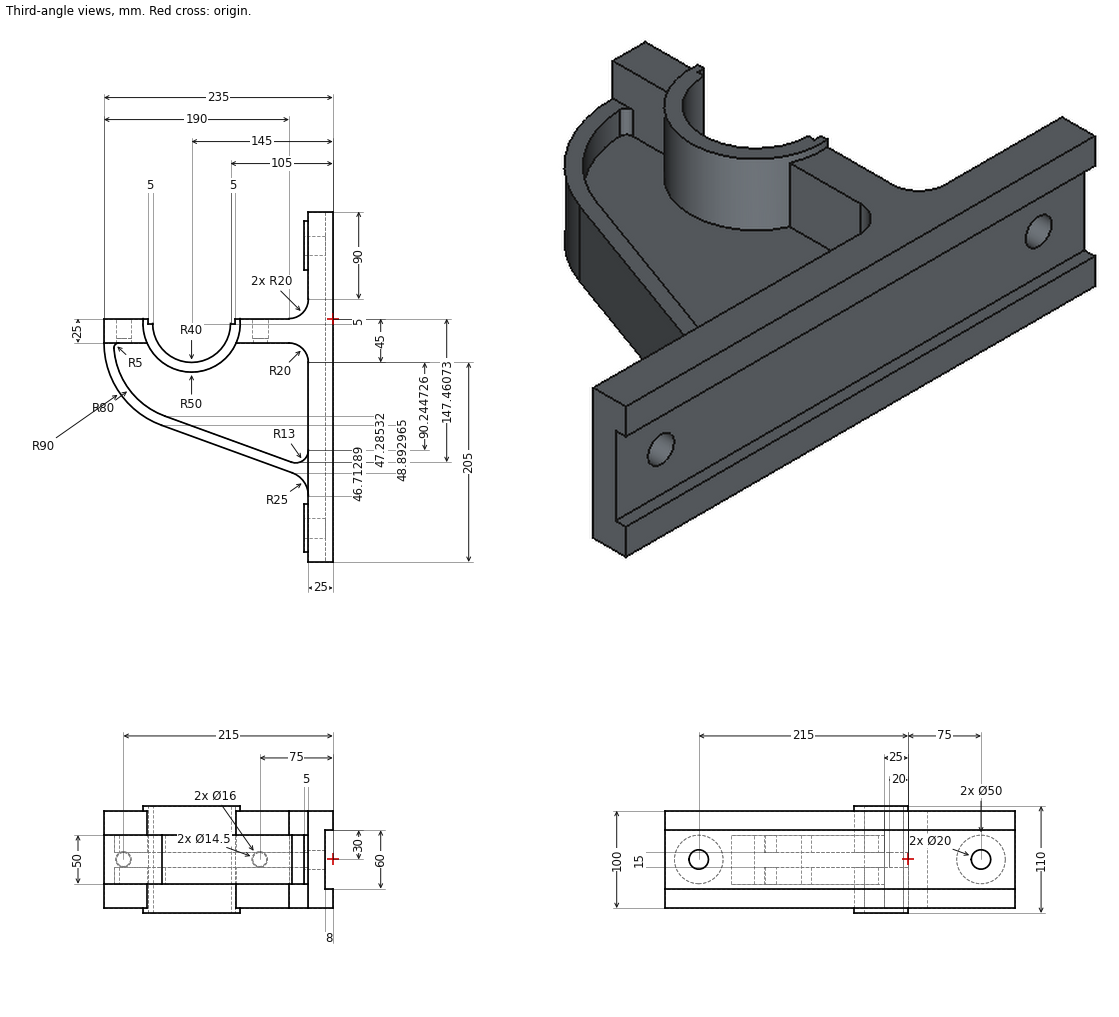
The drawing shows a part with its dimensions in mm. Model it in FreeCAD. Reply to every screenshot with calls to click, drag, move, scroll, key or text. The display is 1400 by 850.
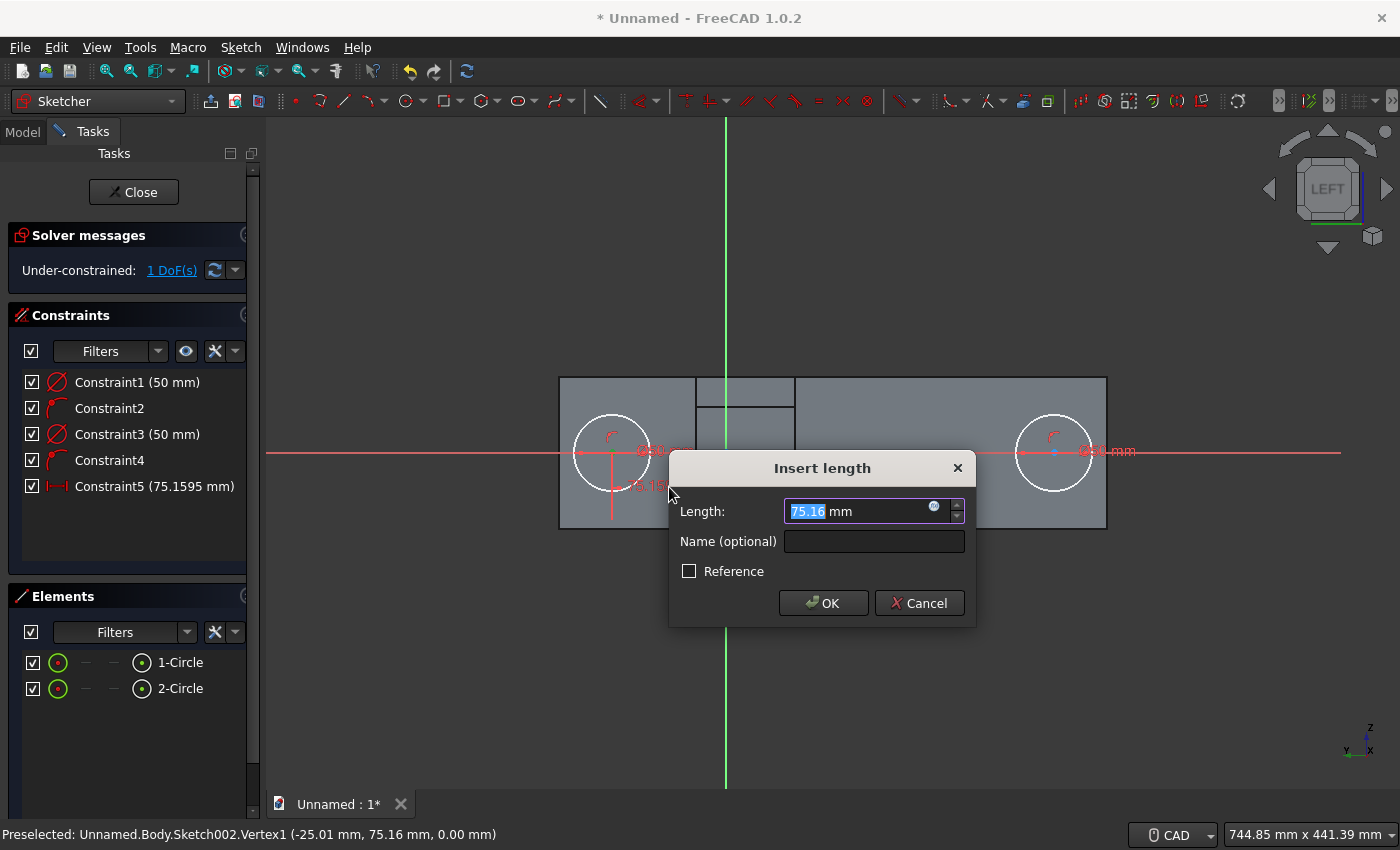
text(75)
key(Return)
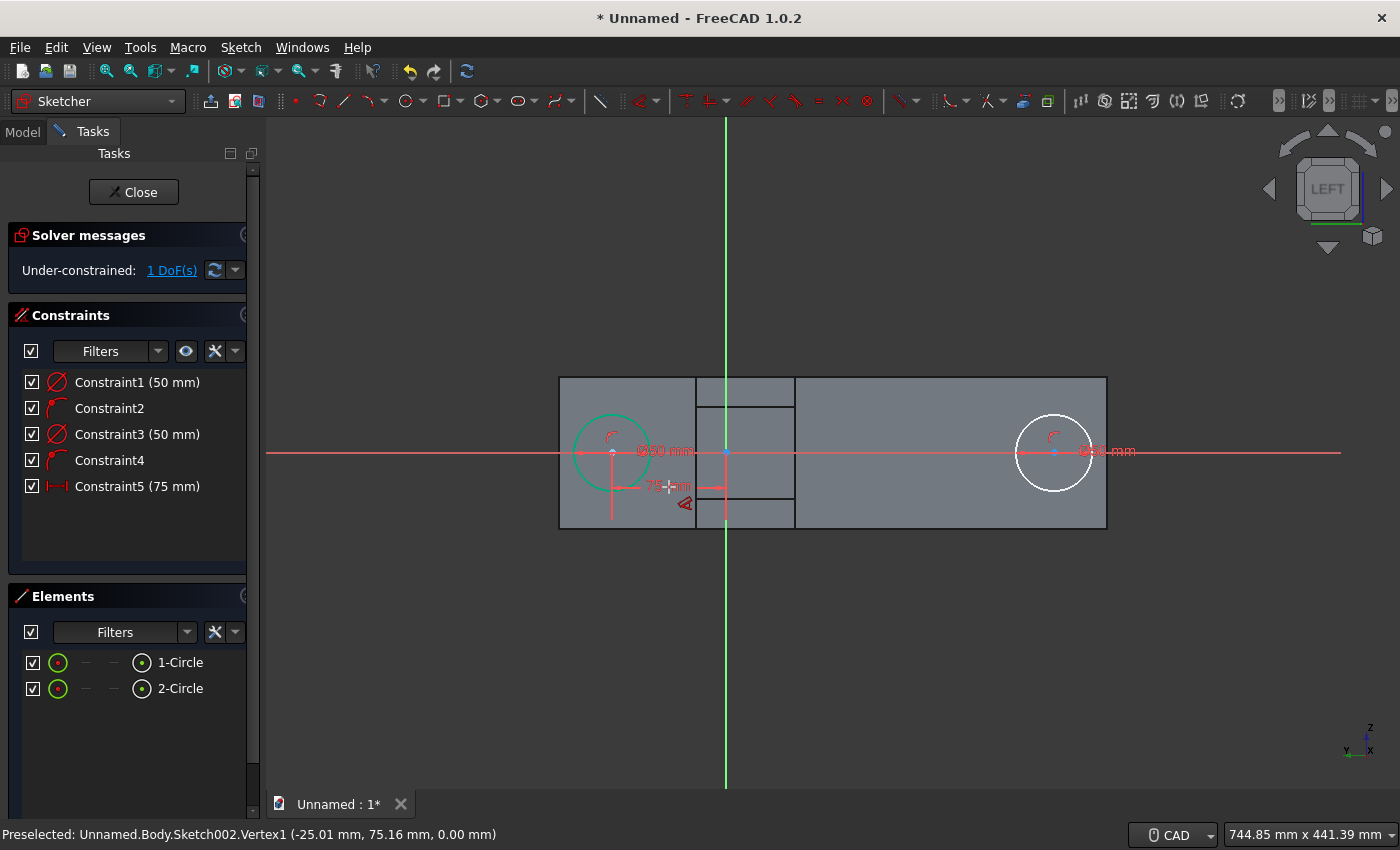
click(1054, 453)
click(890, 487)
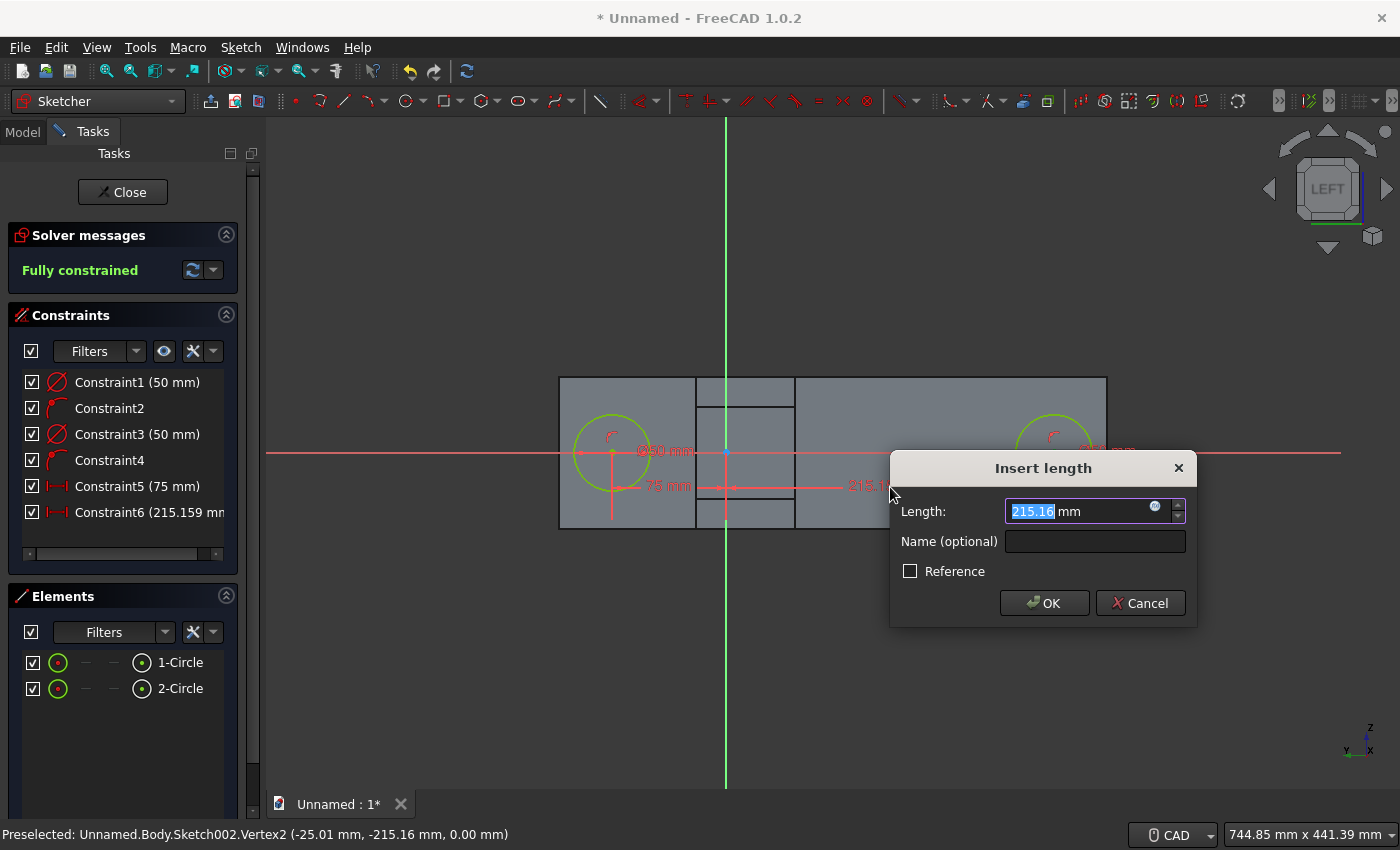
text(215)
key(Return)
key(Escape)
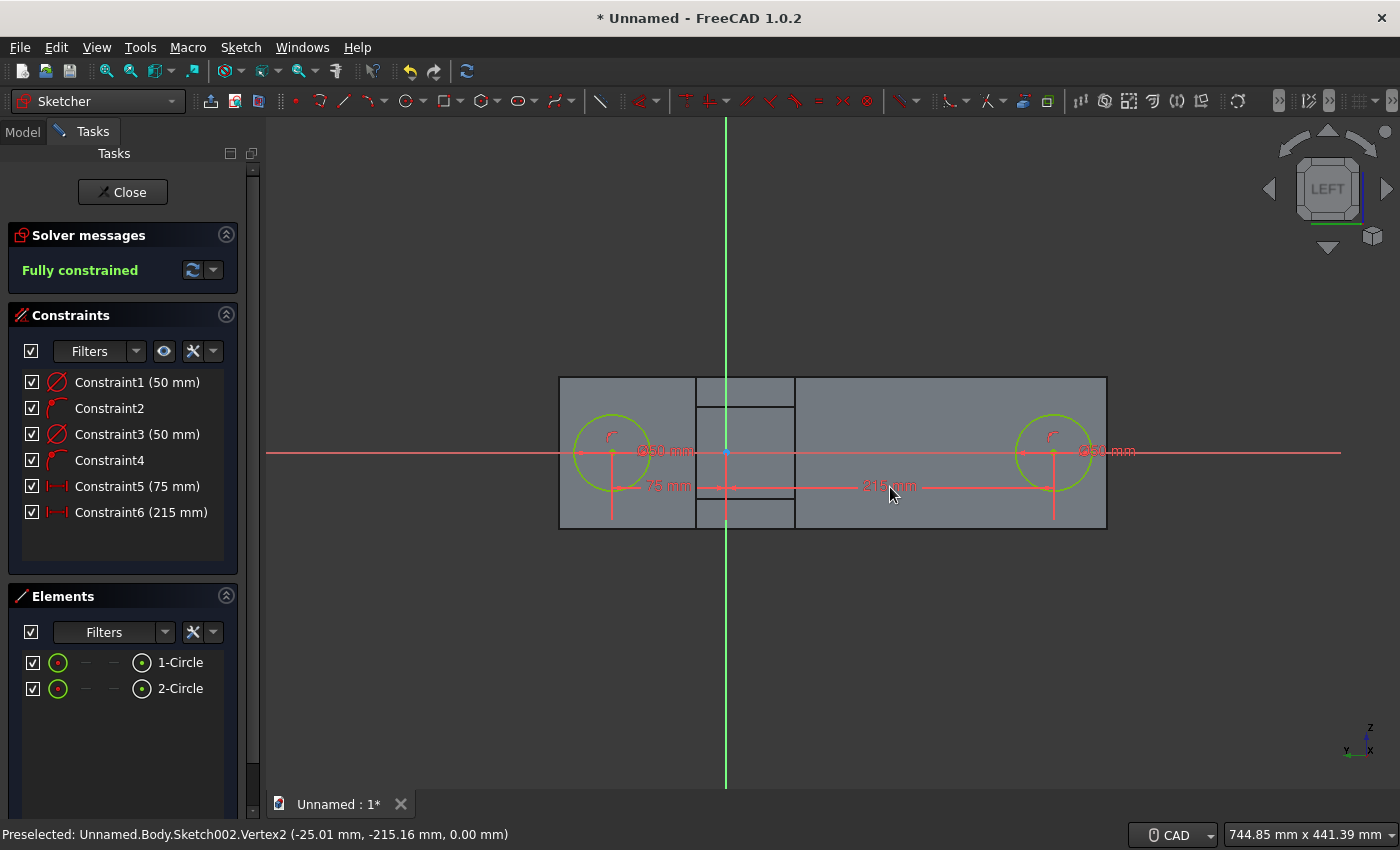
click(123, 192)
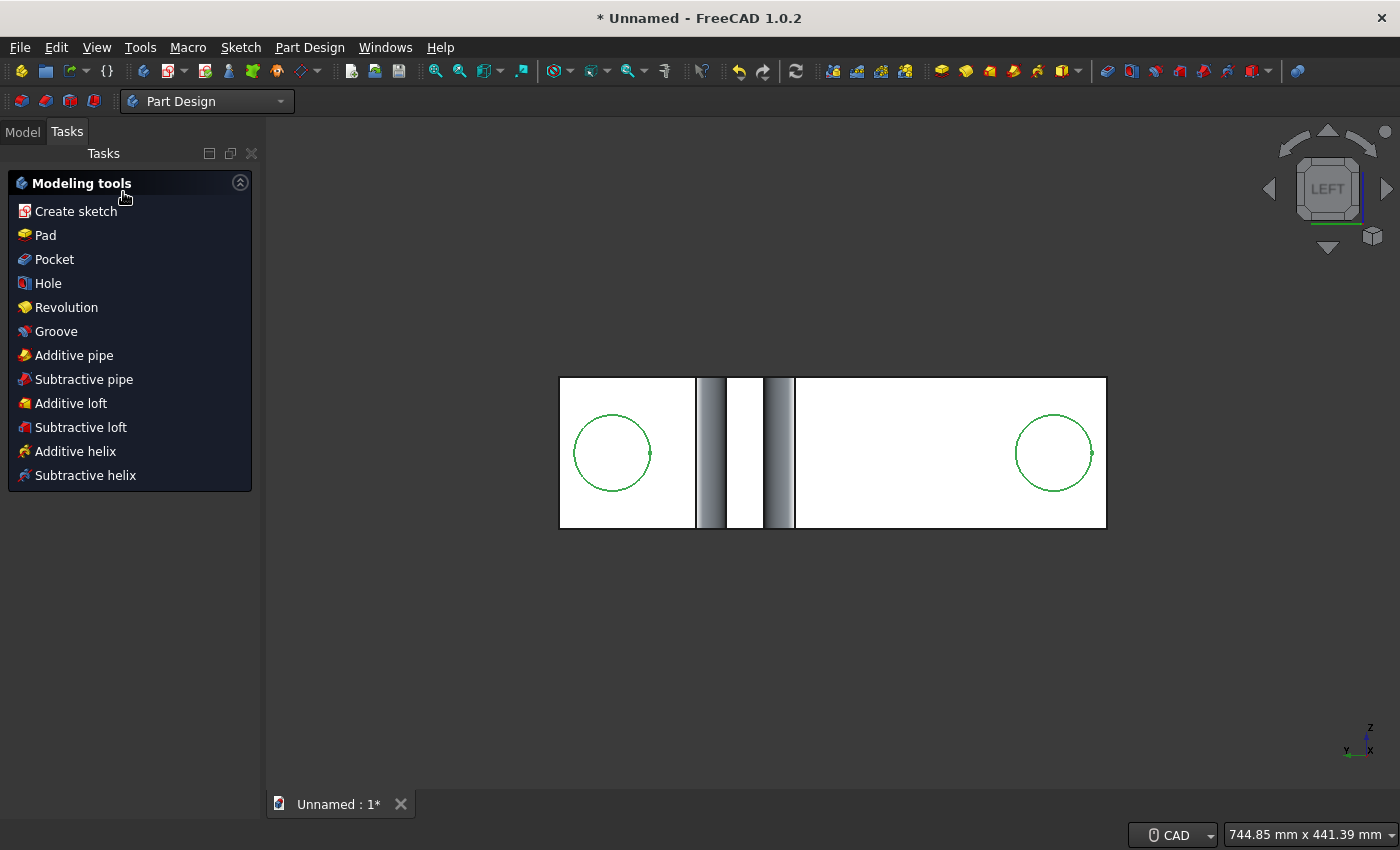
click(942, 72)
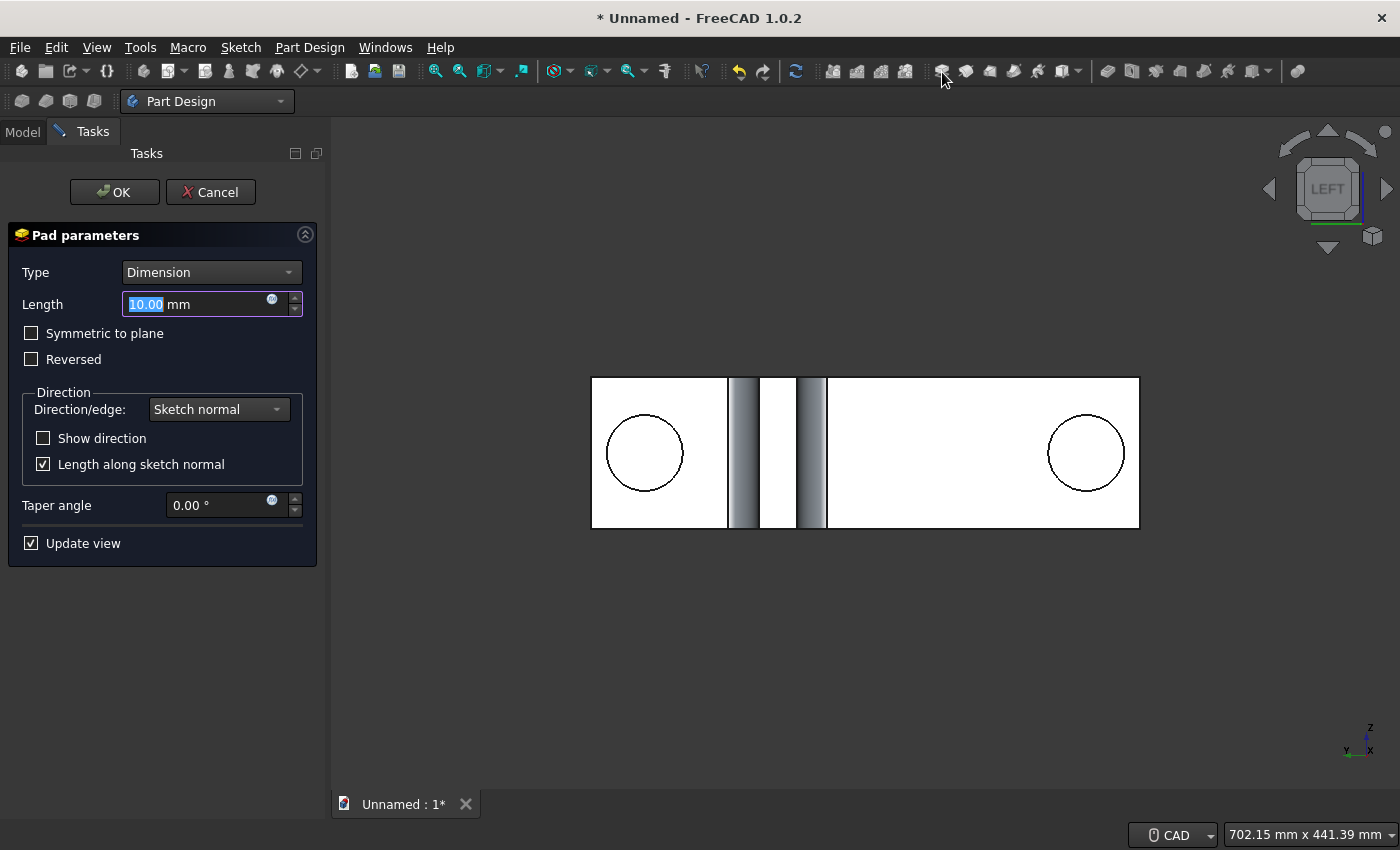
text(5)
key(Tab)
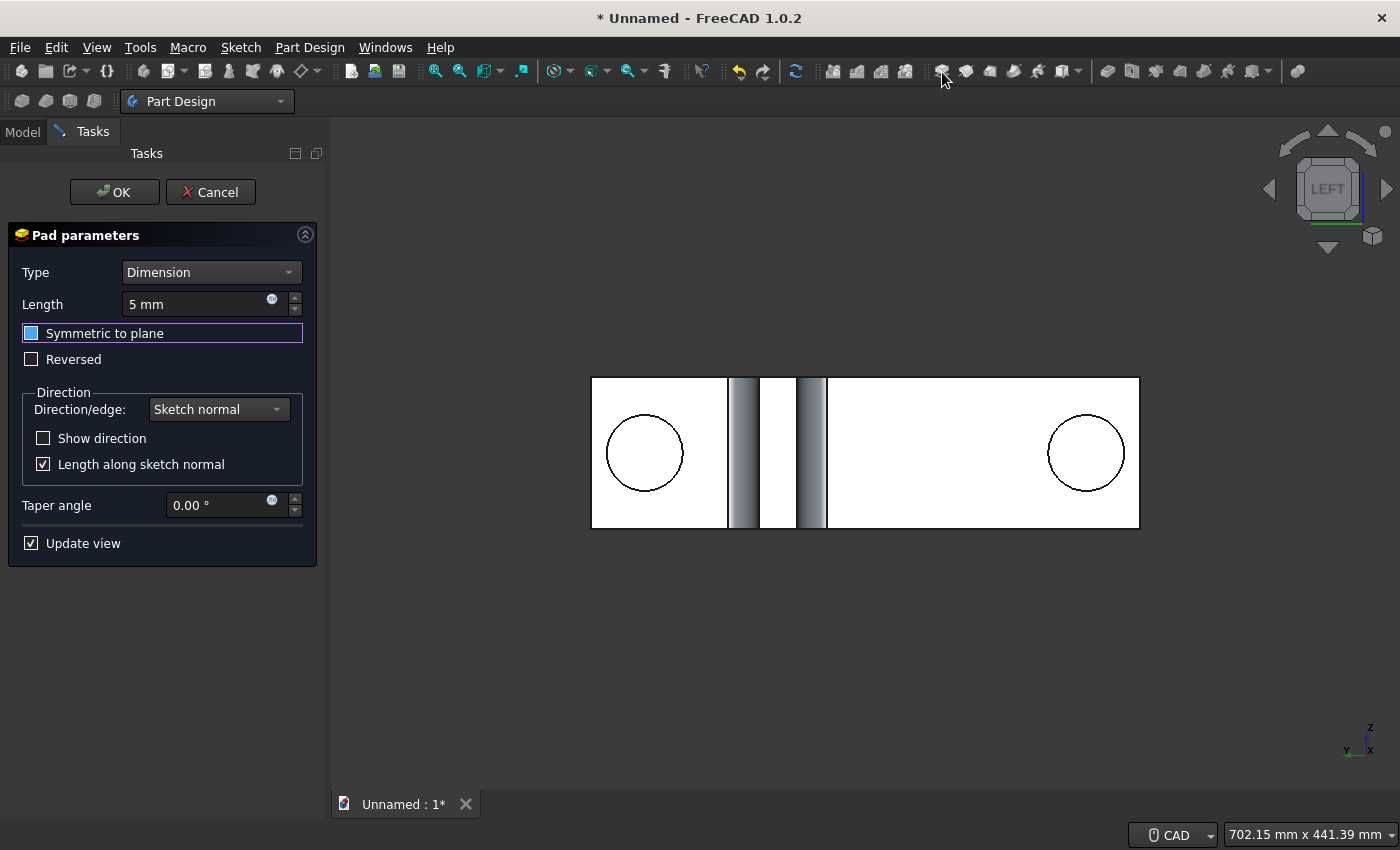
click(115, 192)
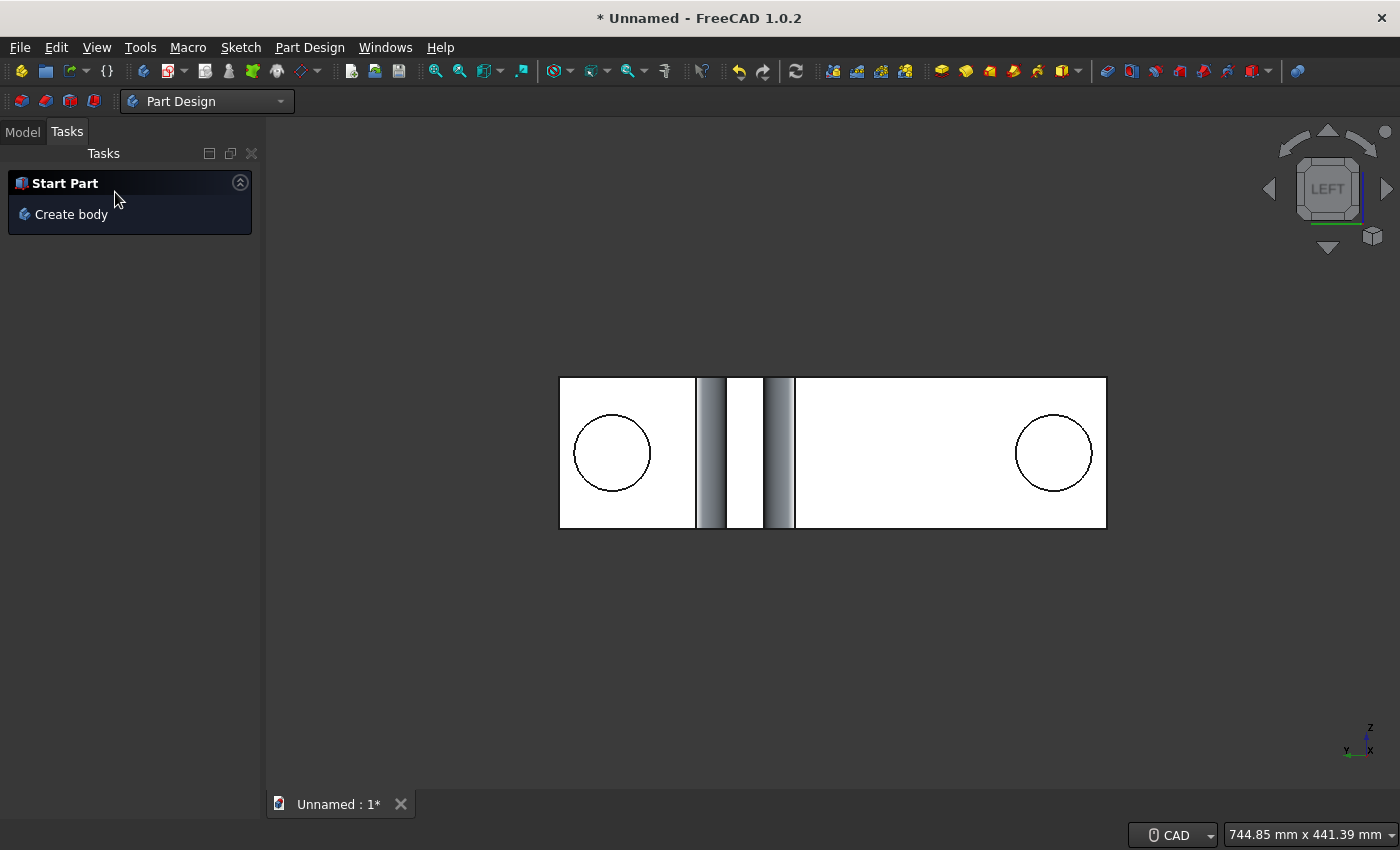
click(1054, 452)